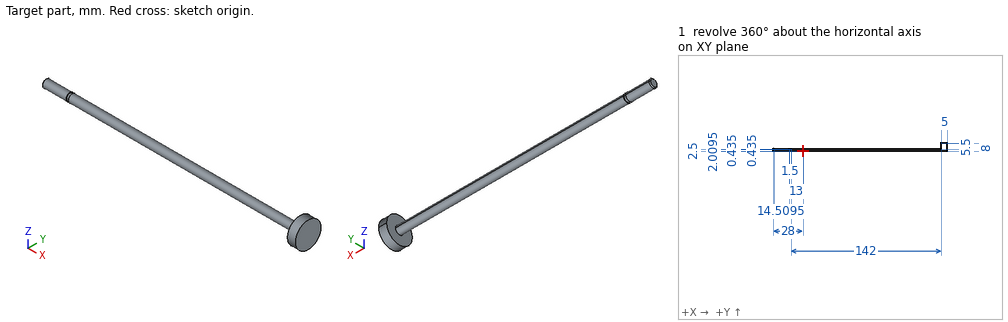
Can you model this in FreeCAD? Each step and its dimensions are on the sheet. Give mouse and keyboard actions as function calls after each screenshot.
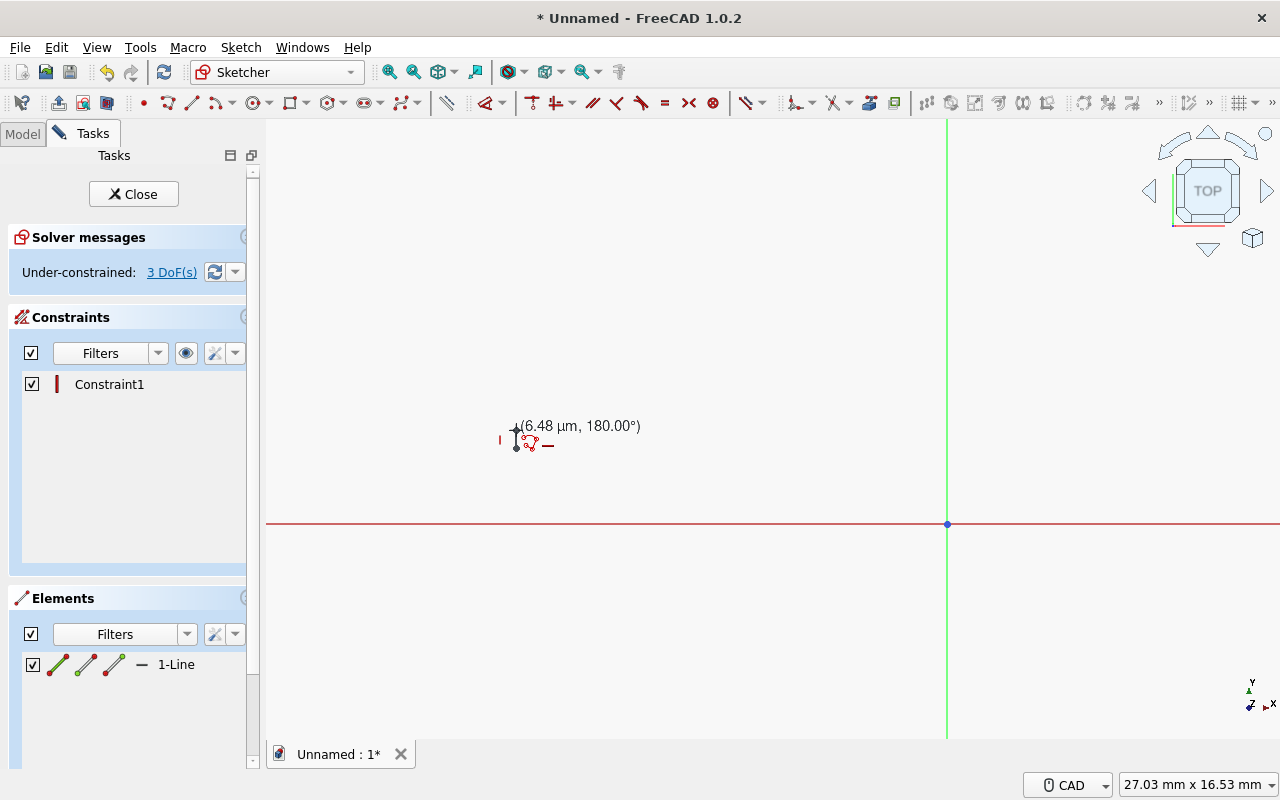
scroll(479, 434, down, 12)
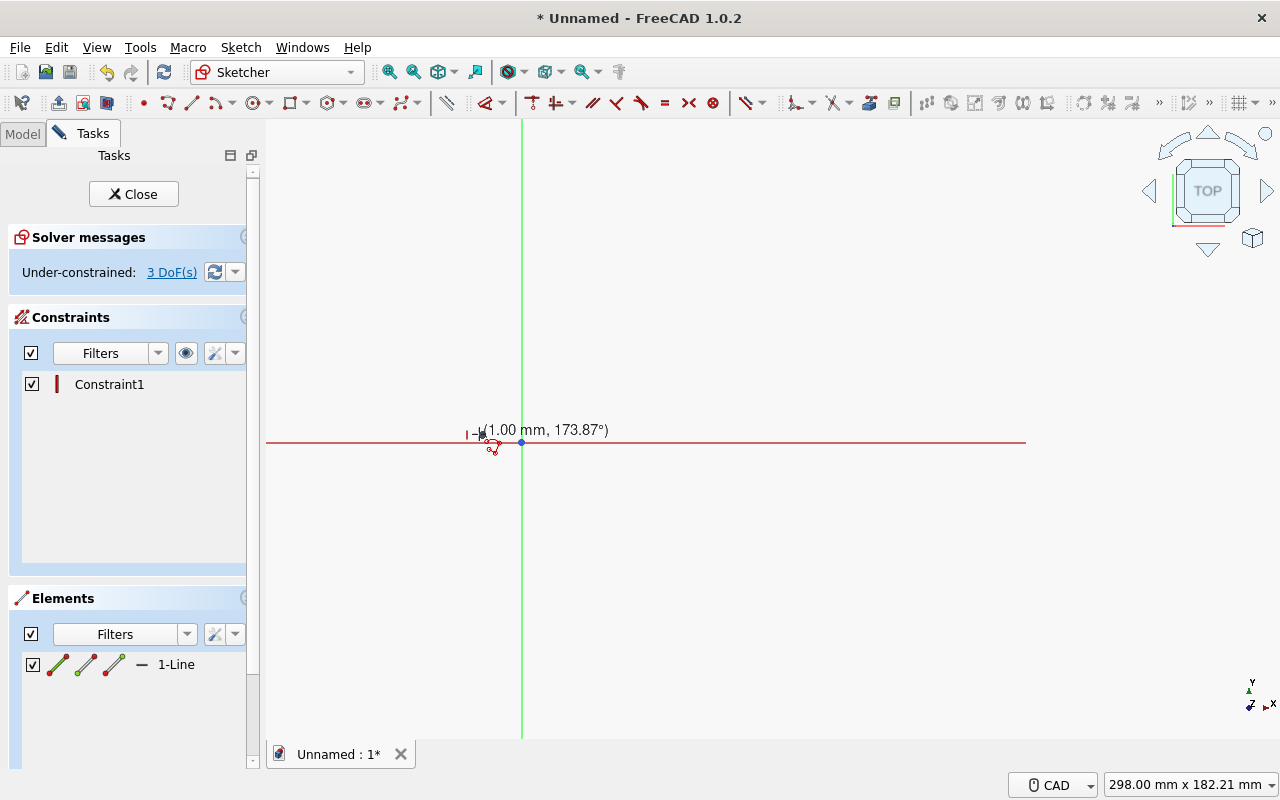
scroll(966, 434, up, 4)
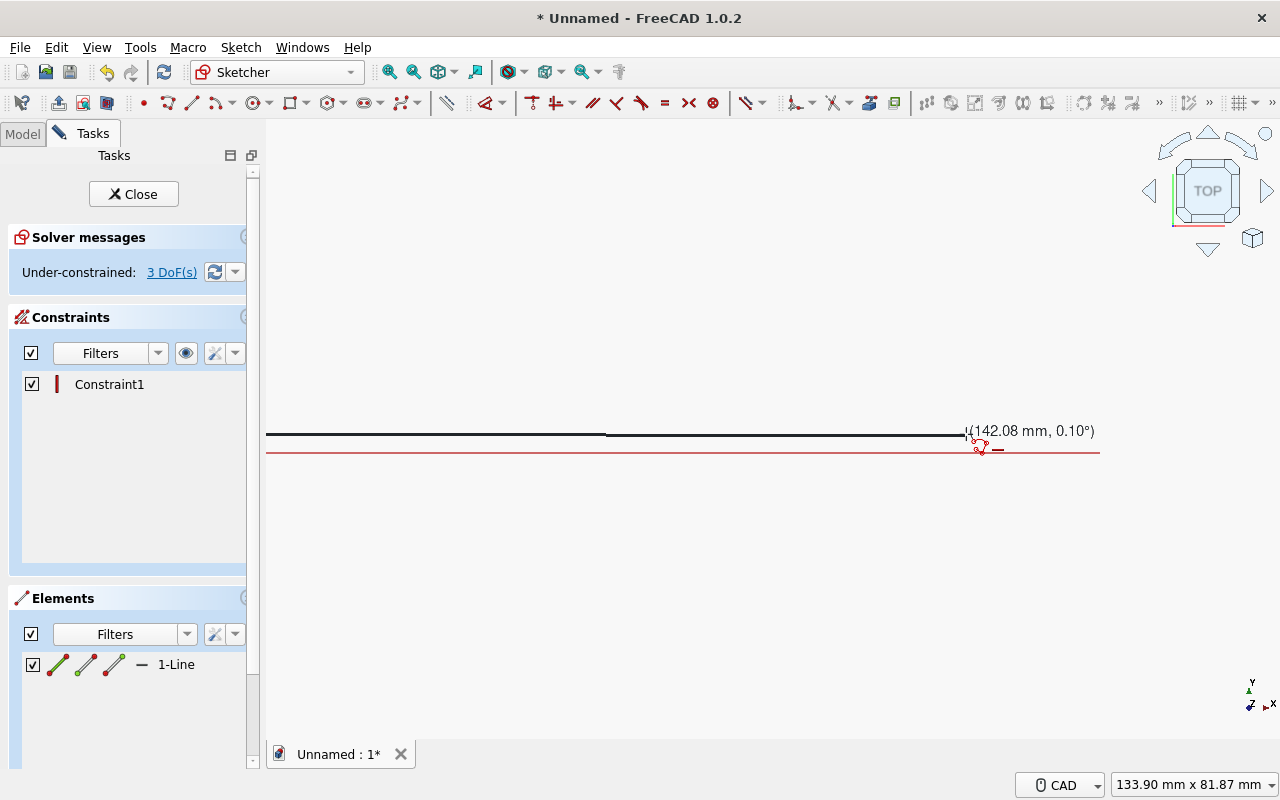
click(965, 434)
click(965, 392)
click(1002, 392)
click(1002, 453)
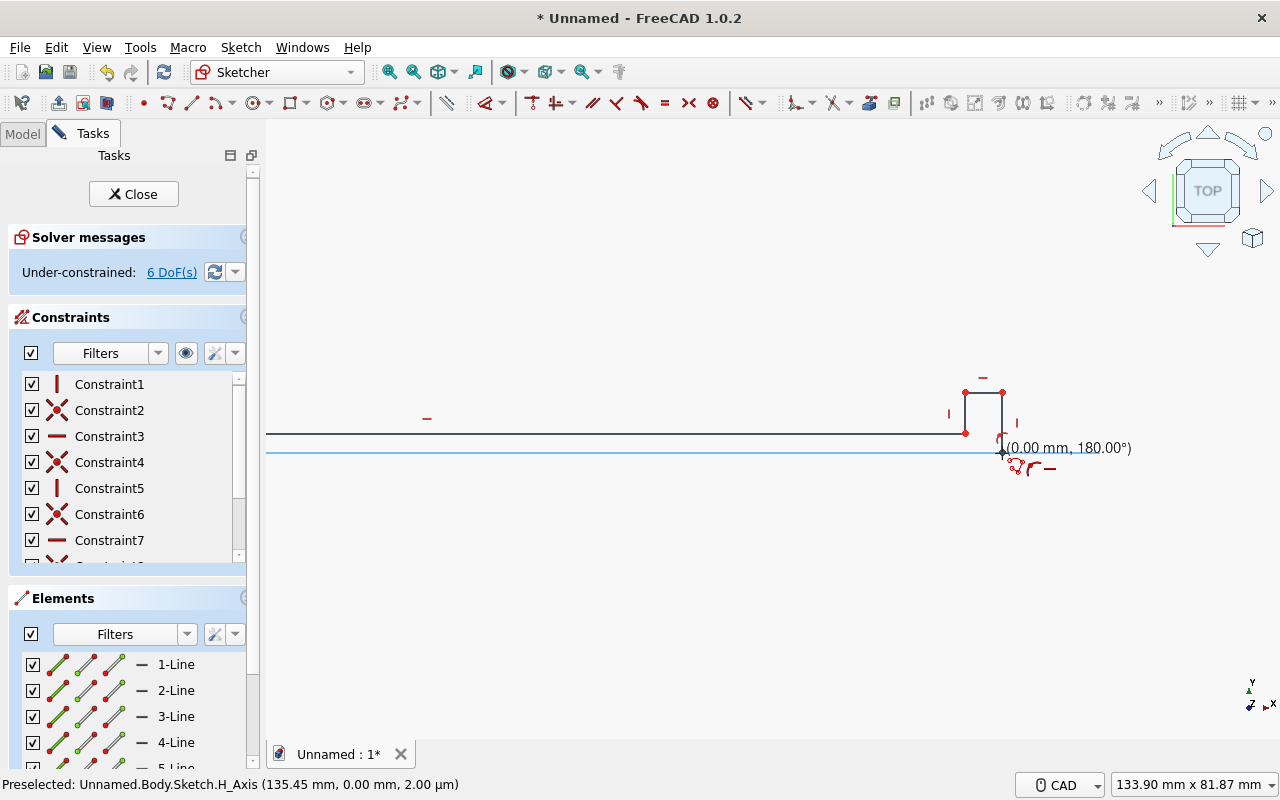
scroll(967, 434, down, 4)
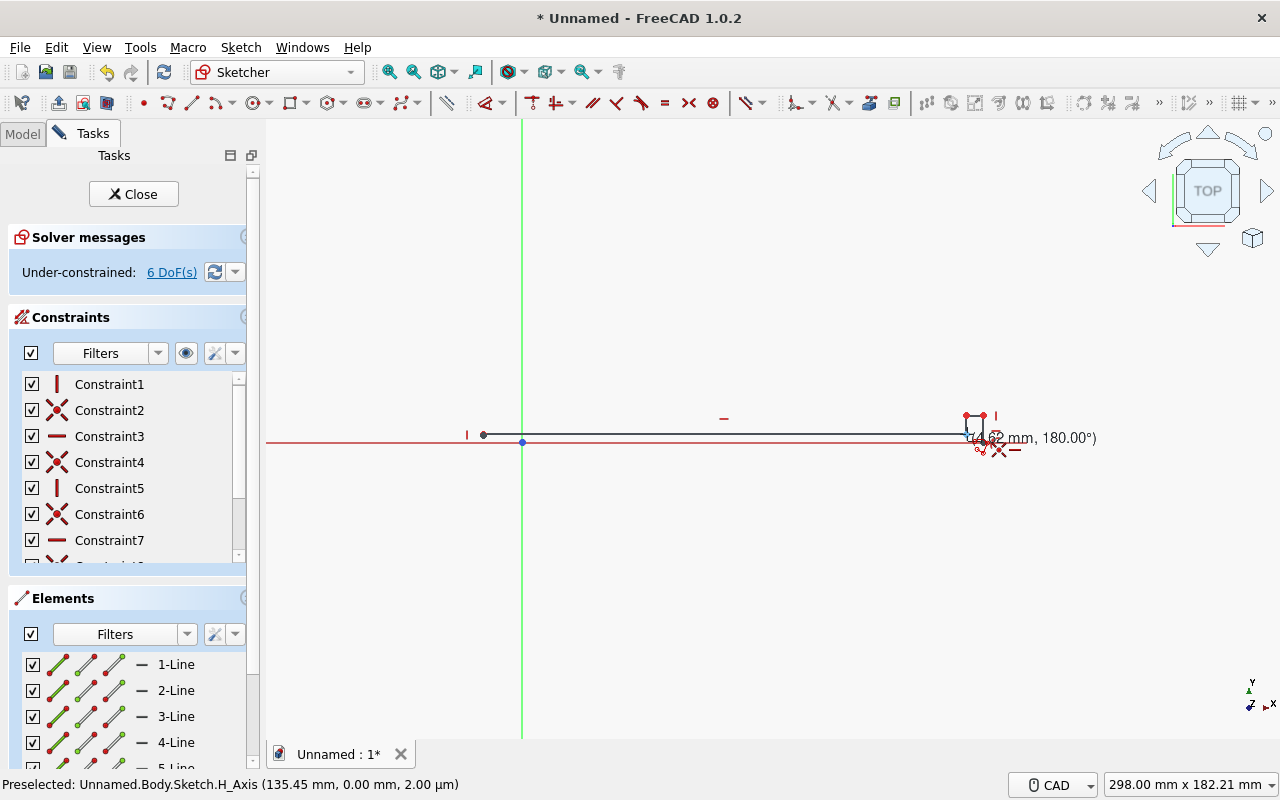
click(427, 434)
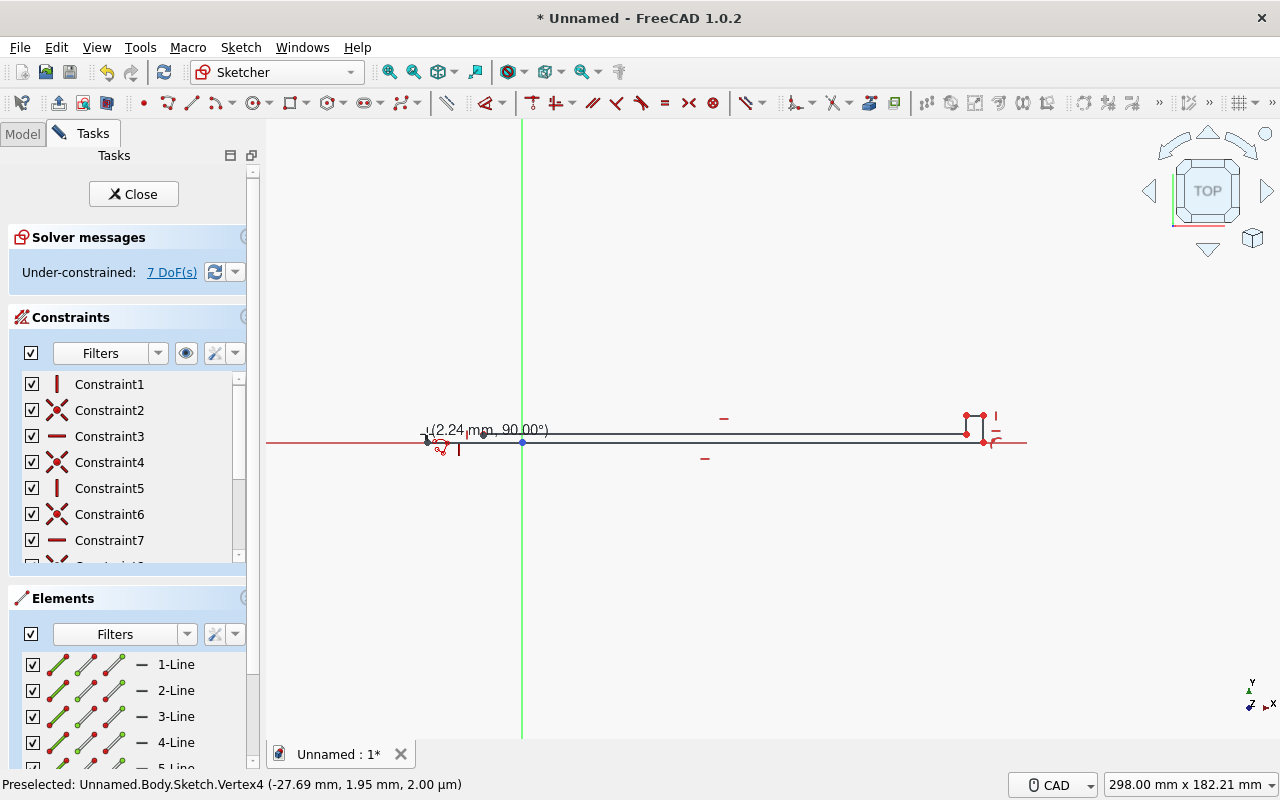
scroll(427, 436, up, 5)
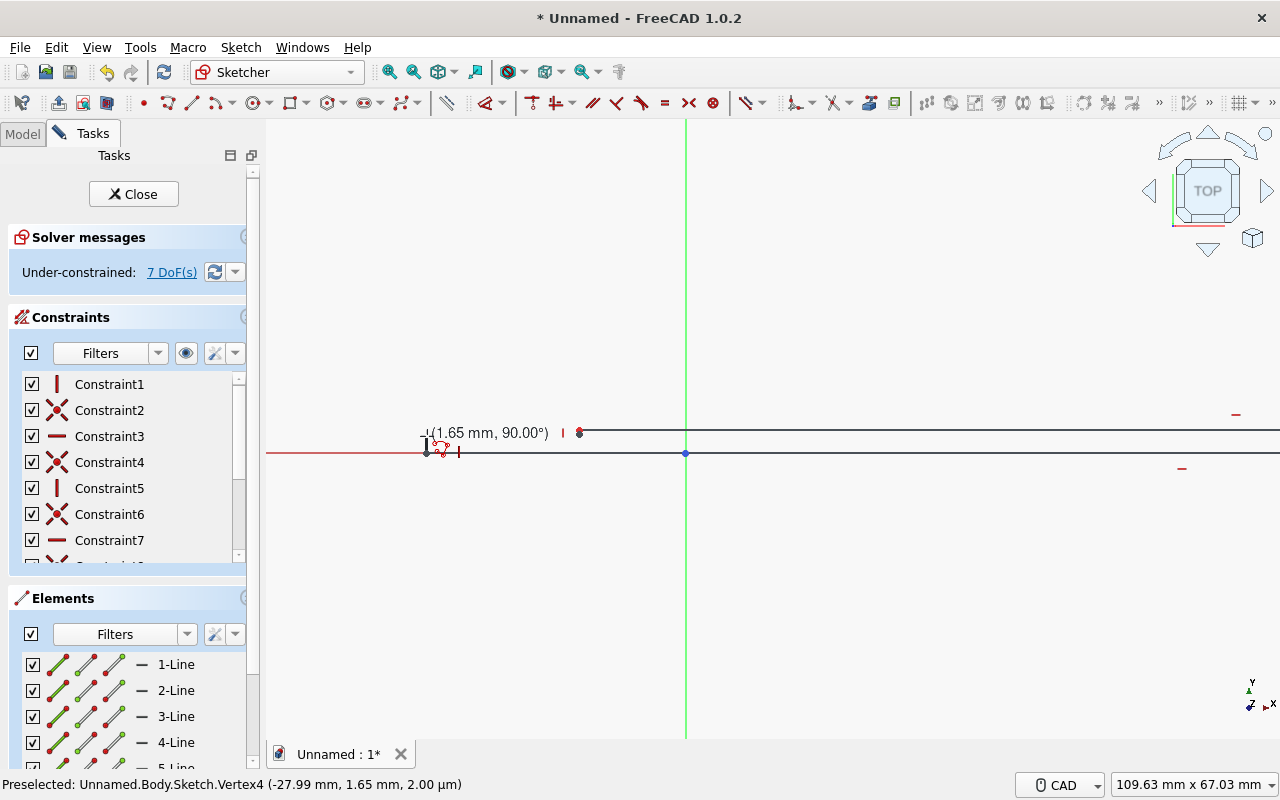
click(427, 435)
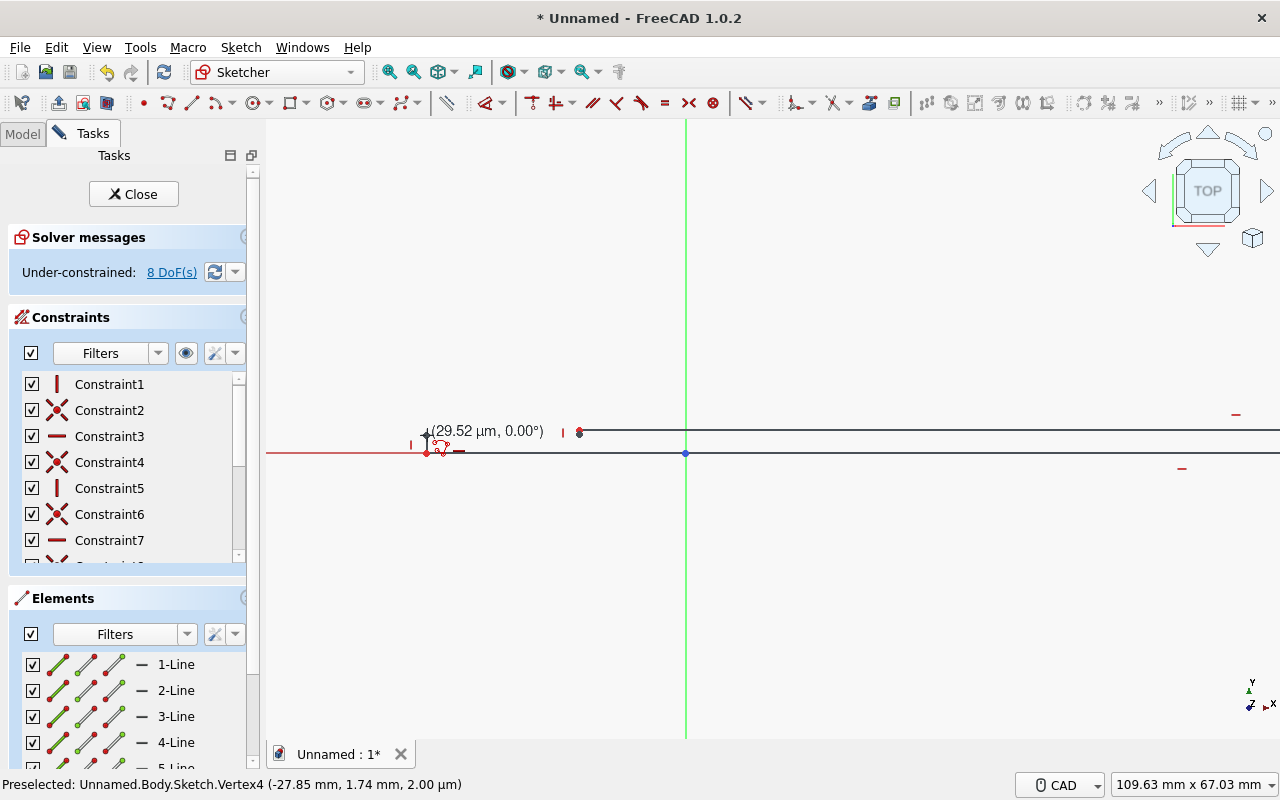
scroll(431, 430, up, 5)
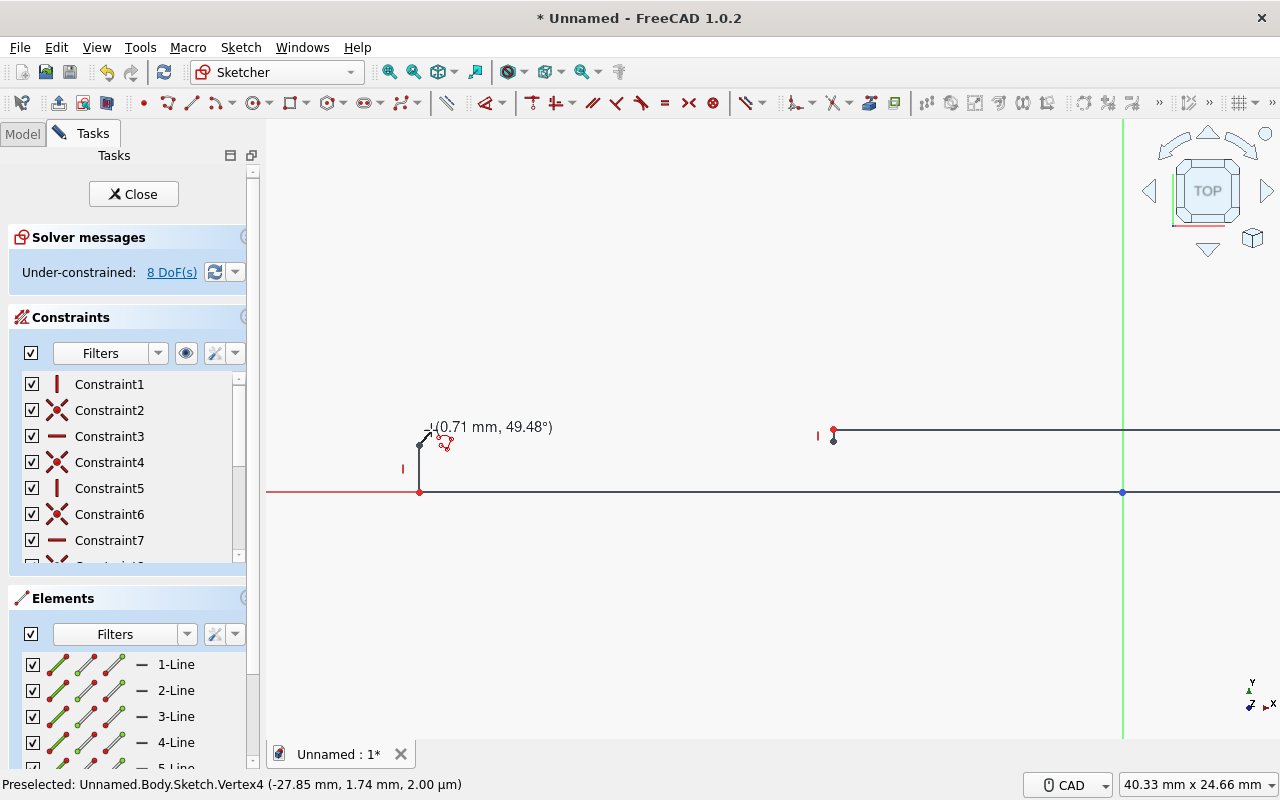
click(431, 429)
click(796, 429)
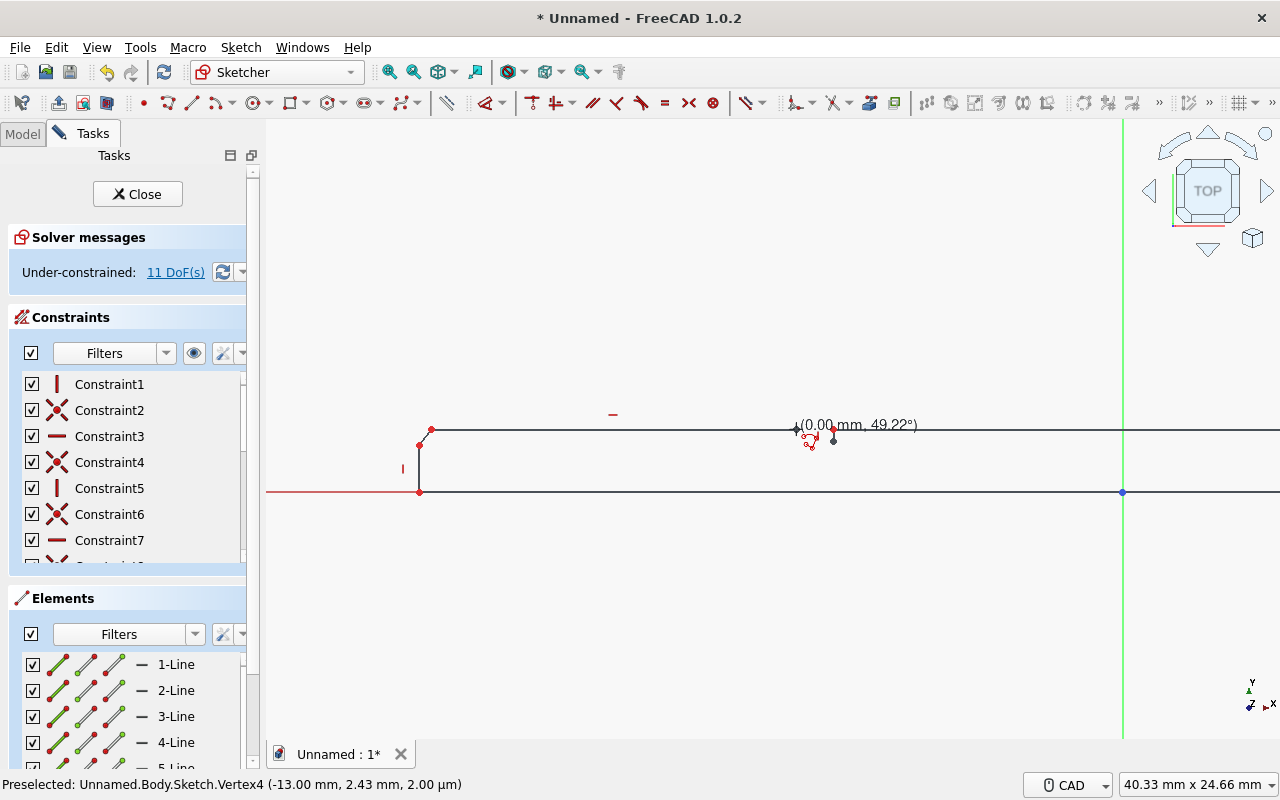
scroll(796, 440, up, 2)